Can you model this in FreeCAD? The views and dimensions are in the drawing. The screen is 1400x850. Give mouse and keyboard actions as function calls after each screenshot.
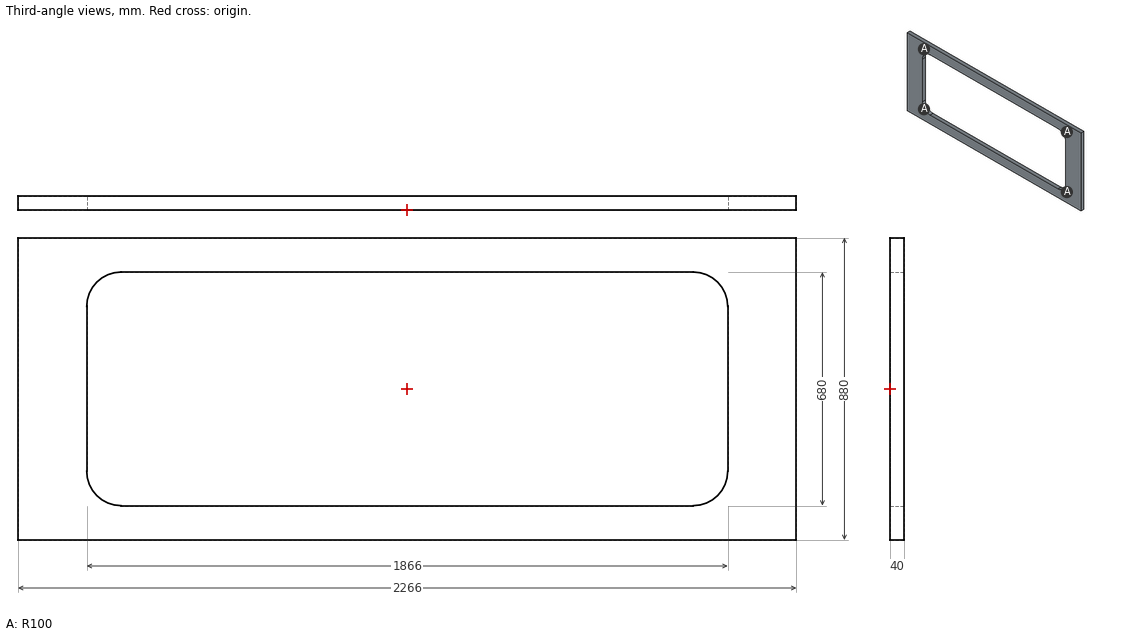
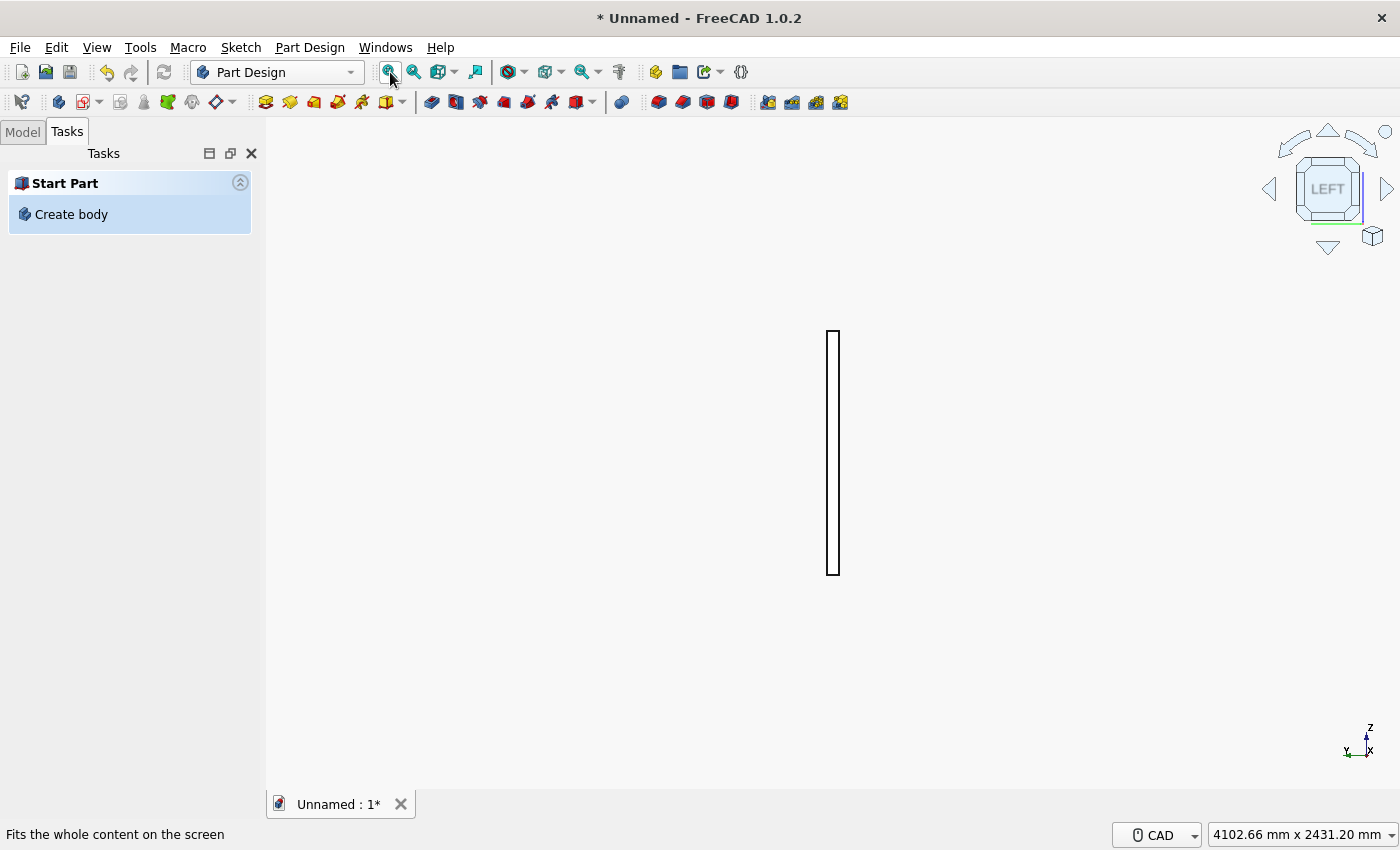
click(390, 72)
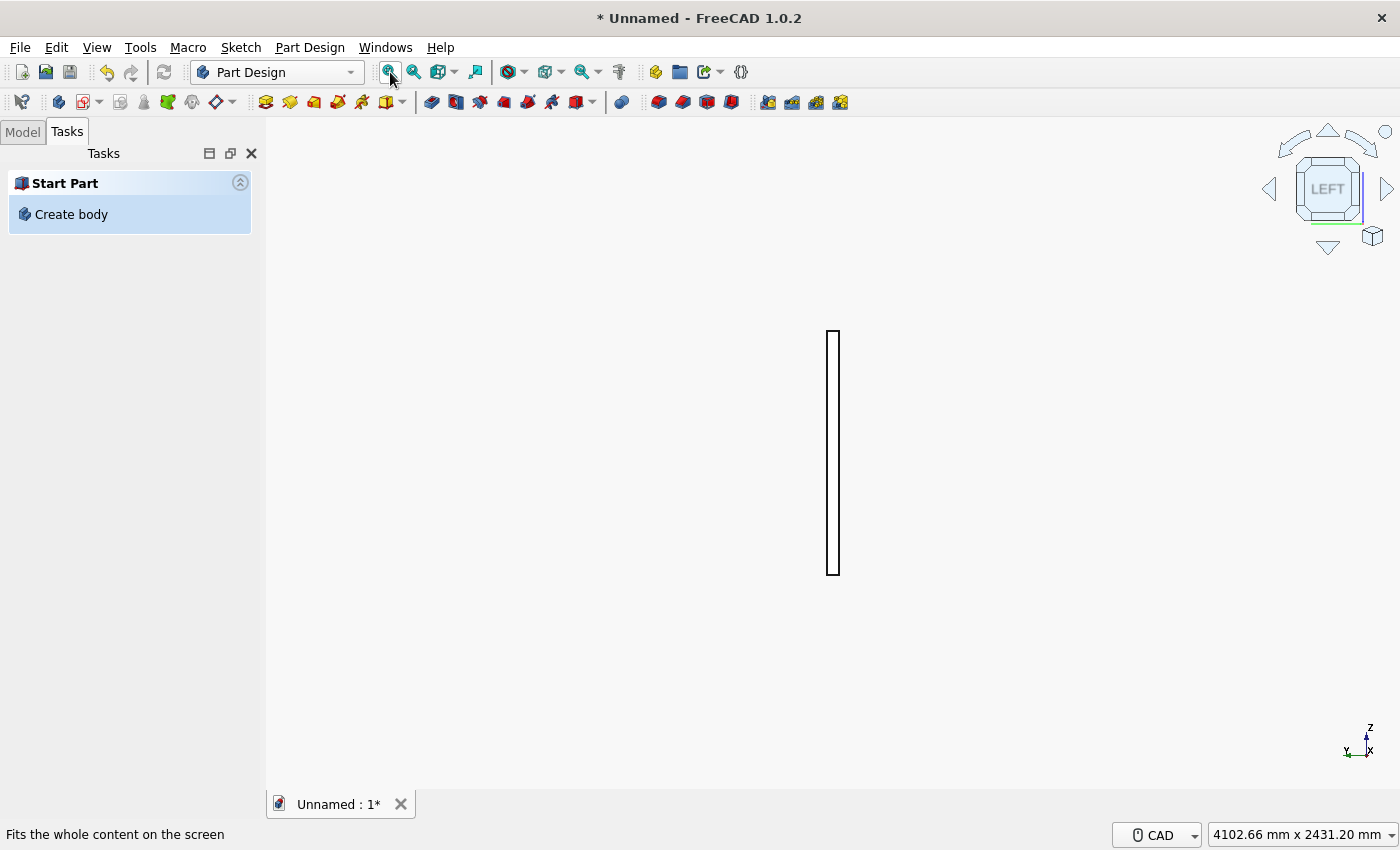
scroll(833, 358, up, 7)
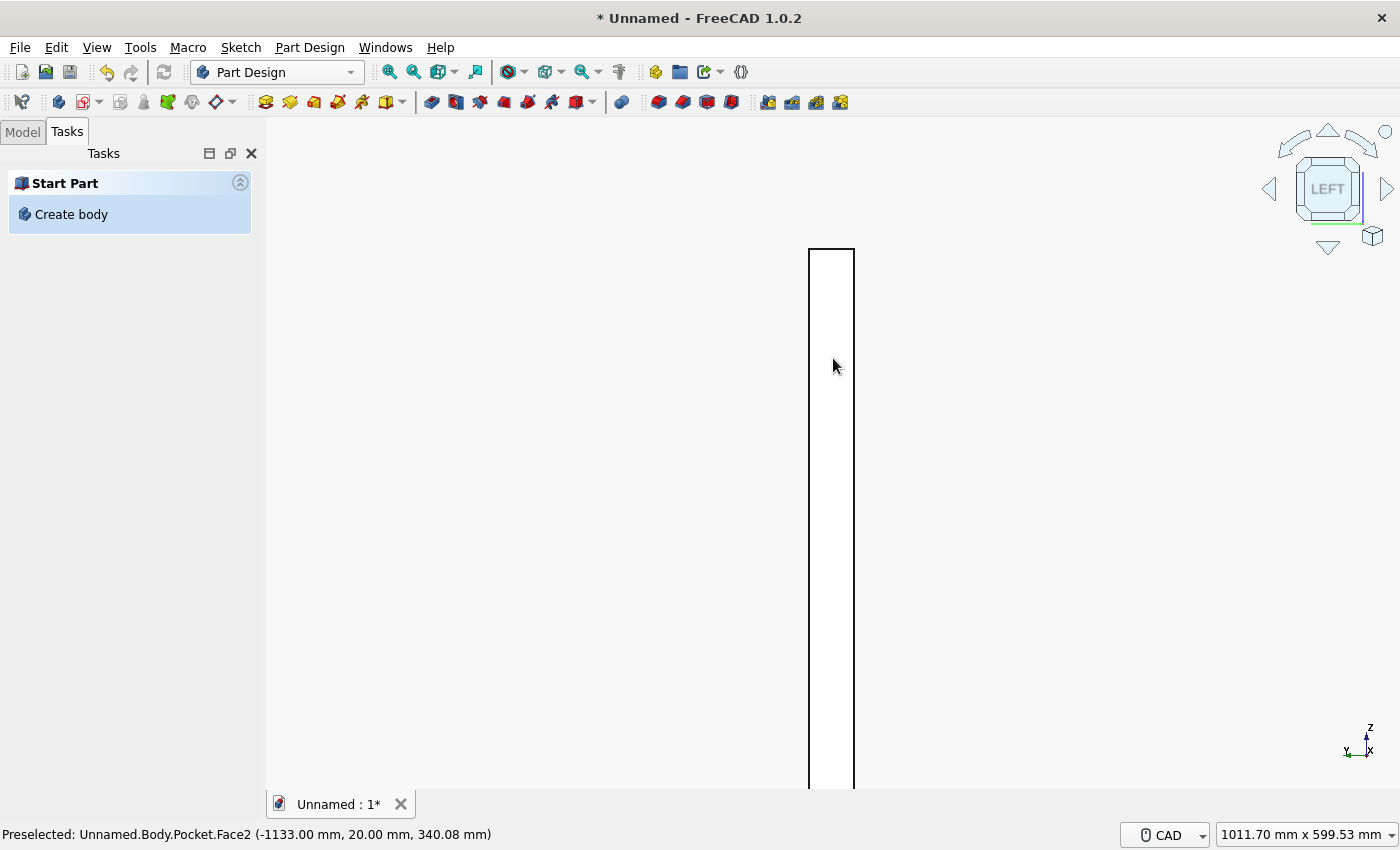
key(v)
key(f)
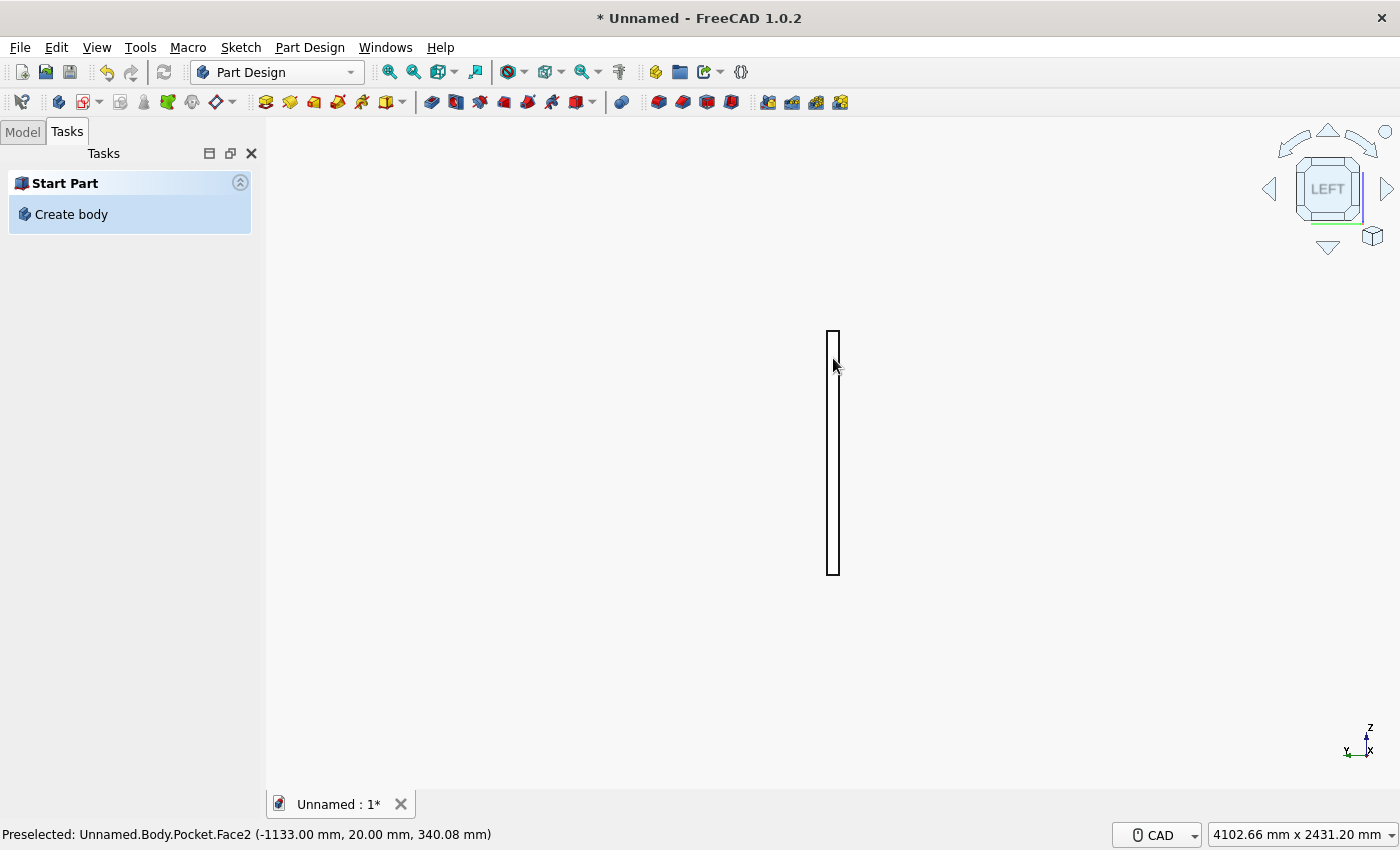
key(v)
key(3)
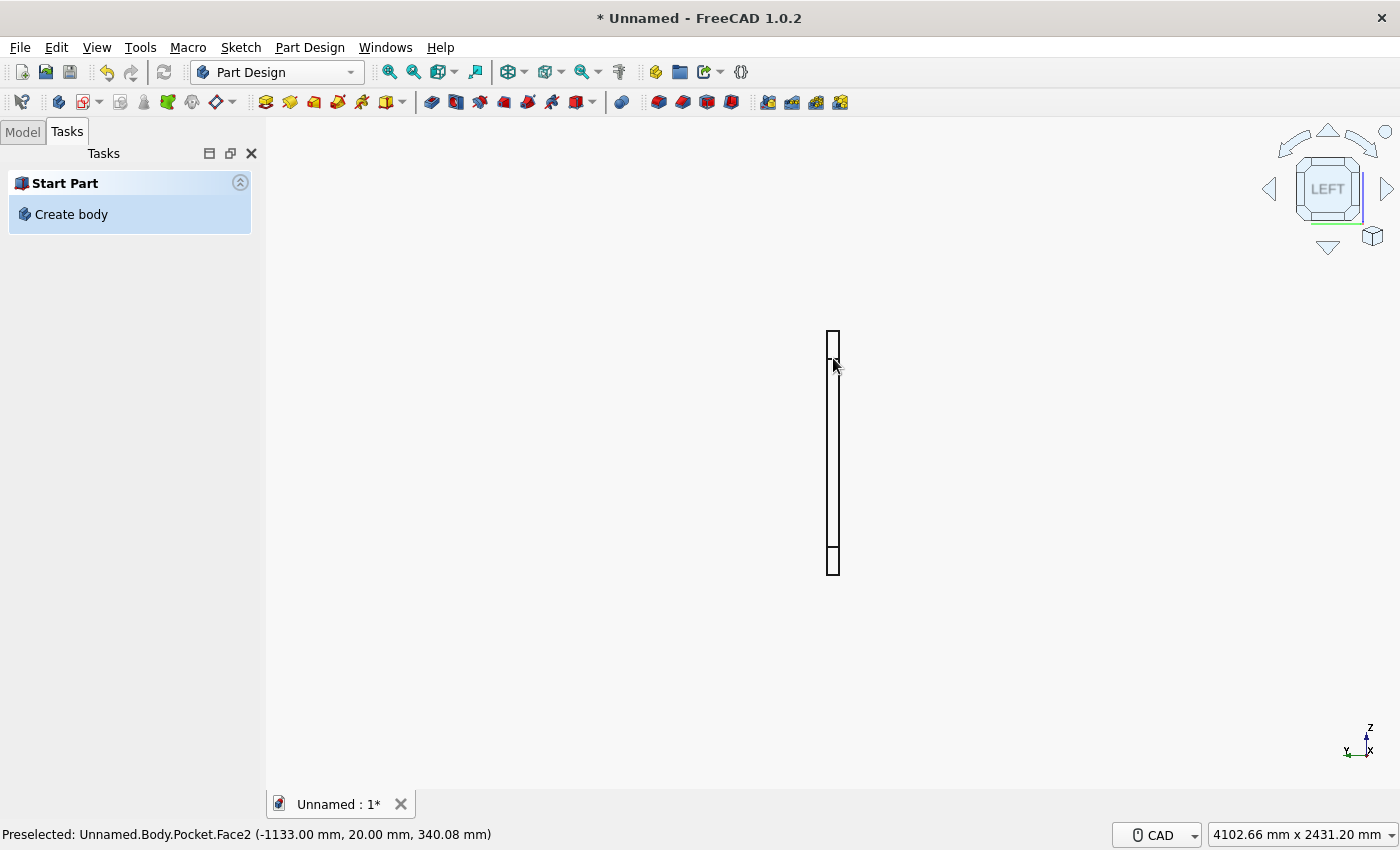
key(0)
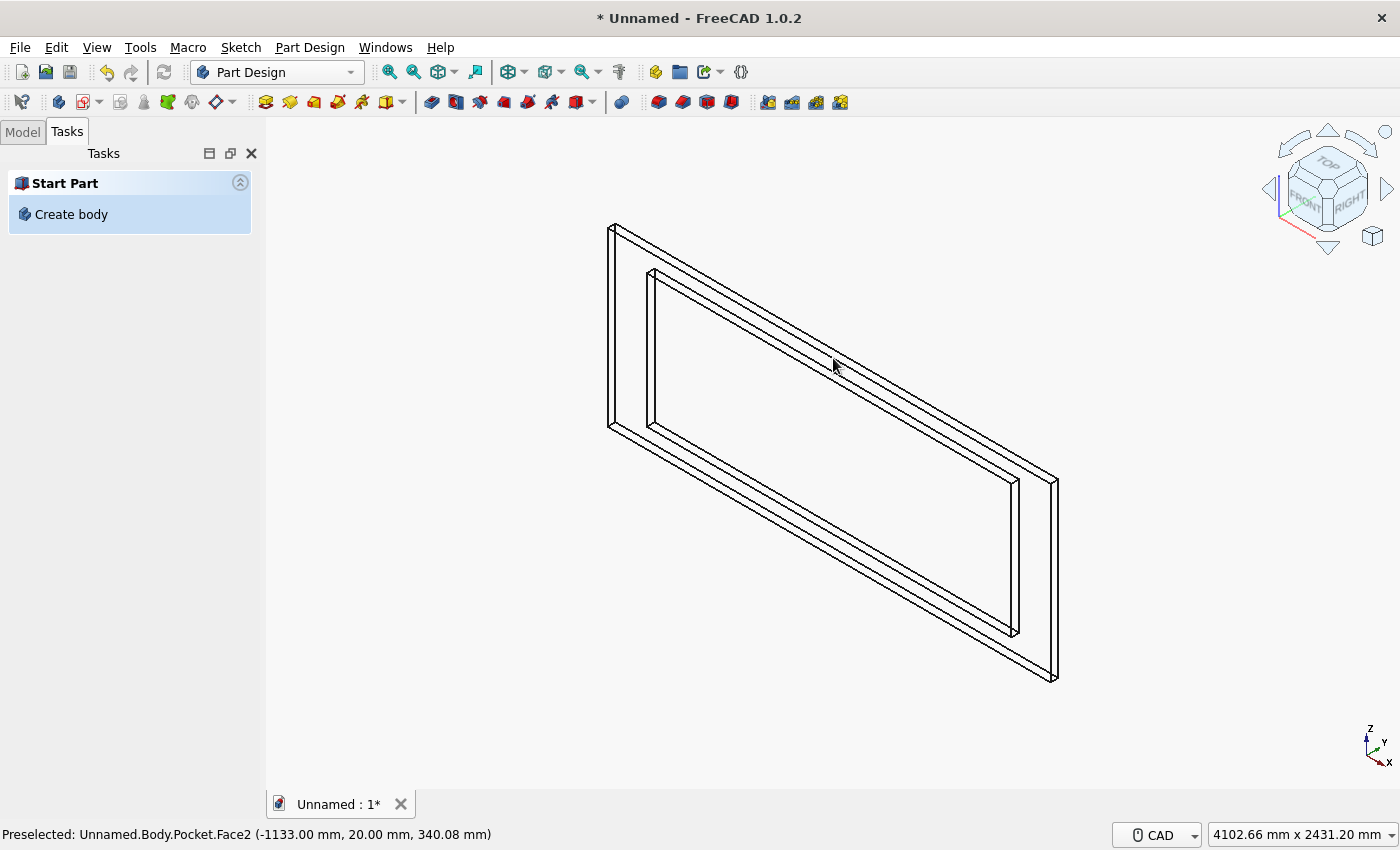
click(1018, 479)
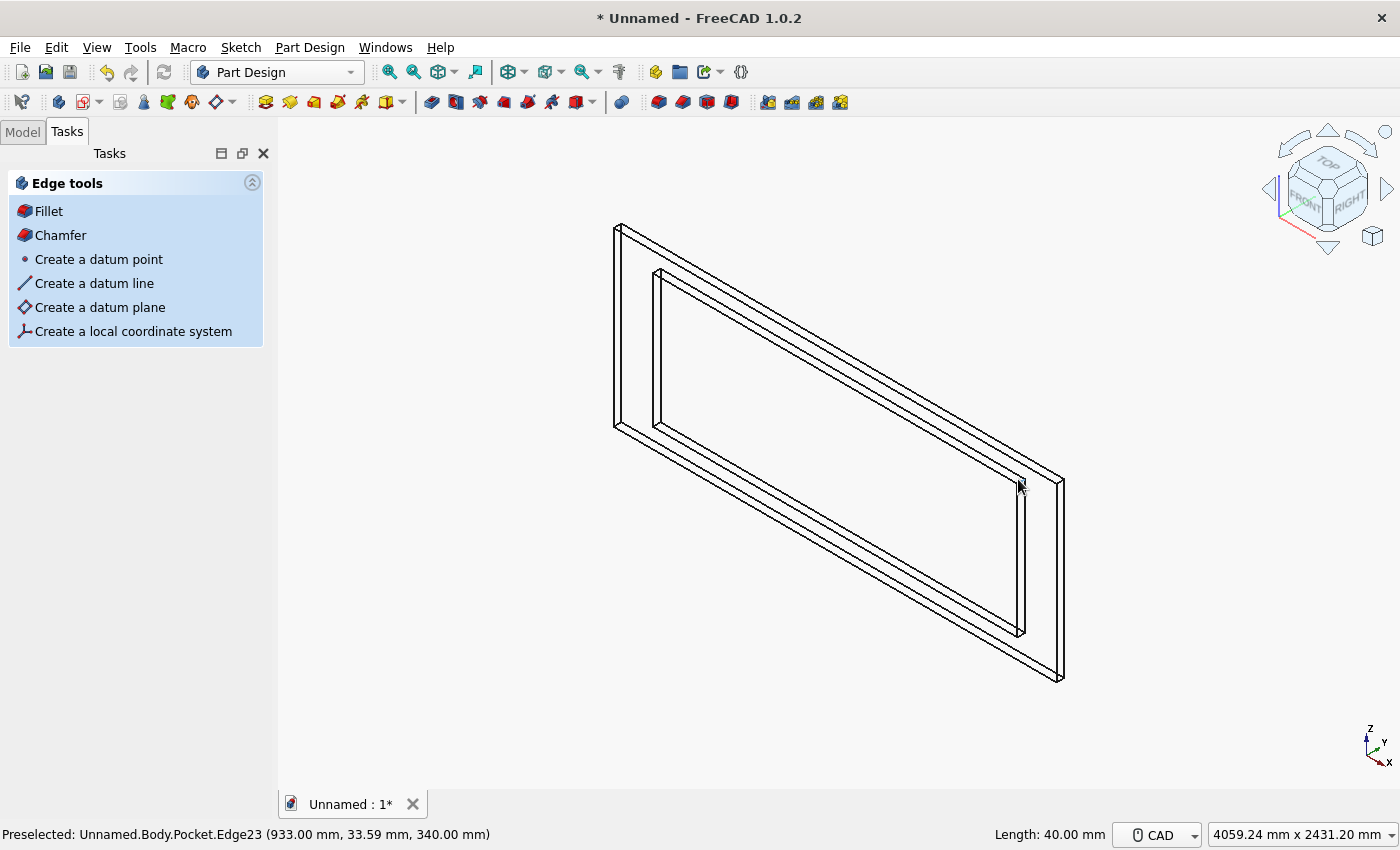
click(1024, 633, ctrl)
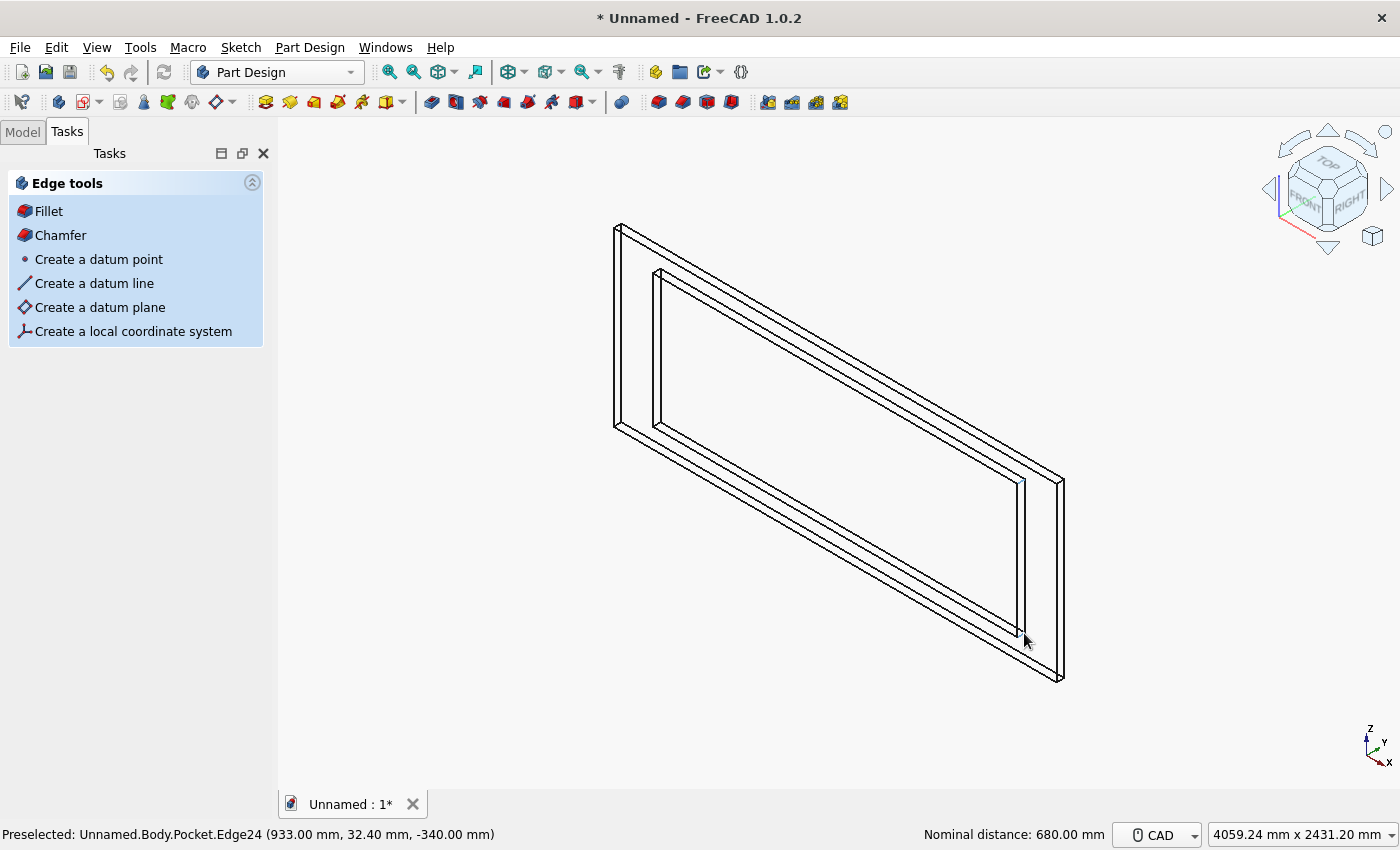
scroll(657, 423, up, 7)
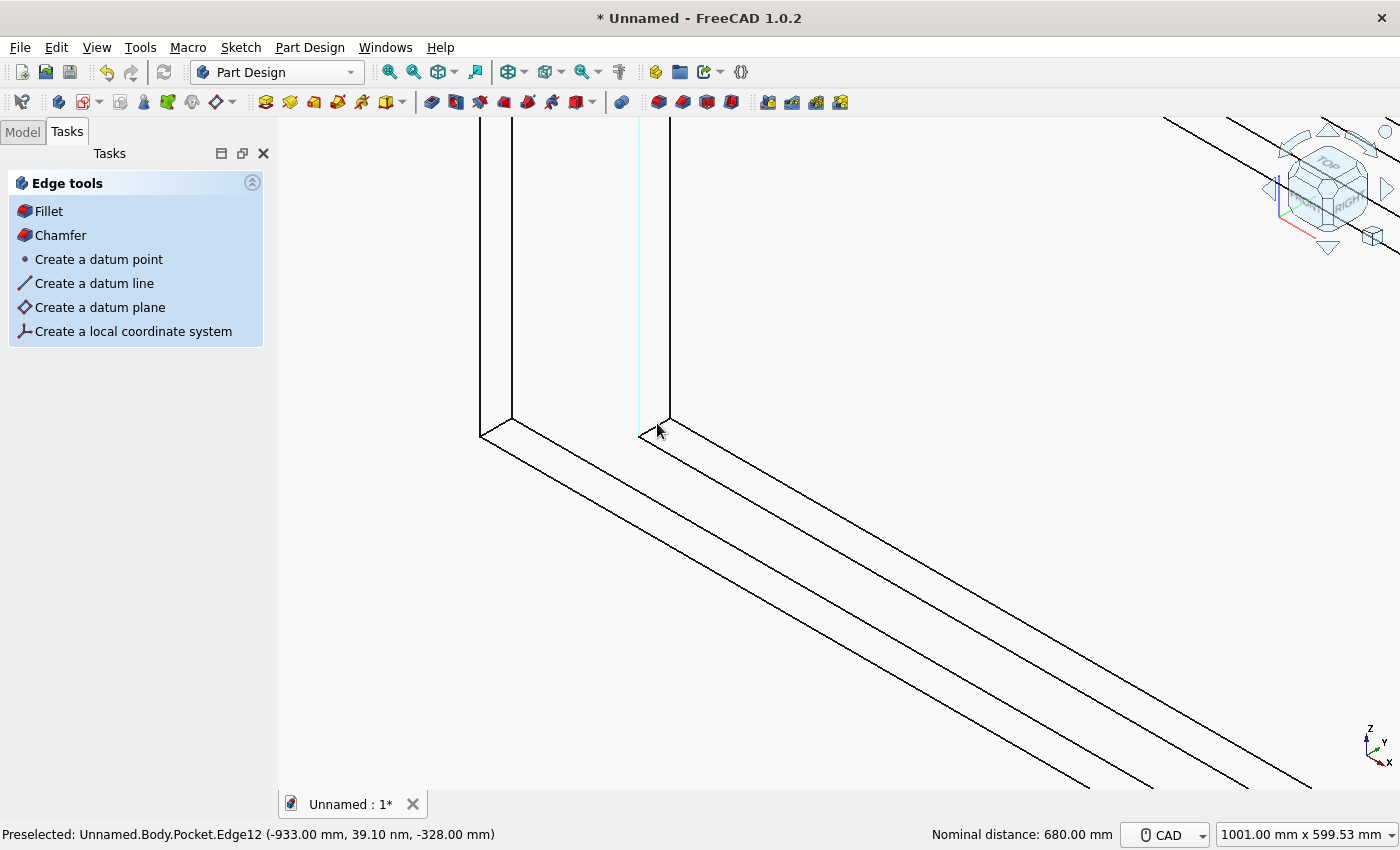
click(655, 426, ctrl)